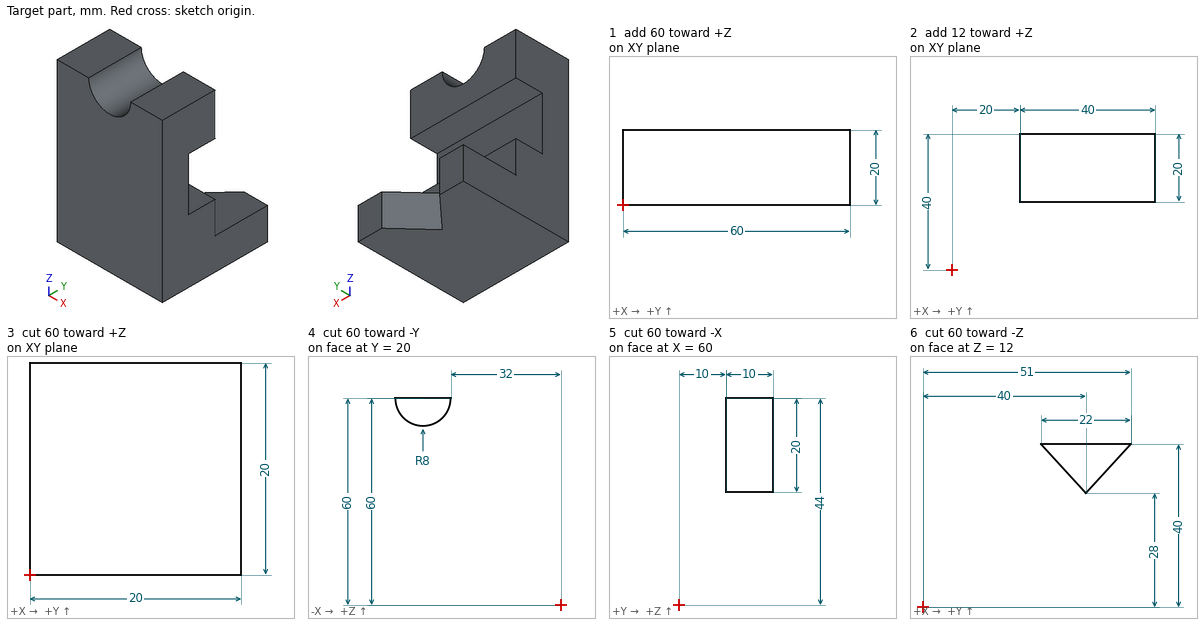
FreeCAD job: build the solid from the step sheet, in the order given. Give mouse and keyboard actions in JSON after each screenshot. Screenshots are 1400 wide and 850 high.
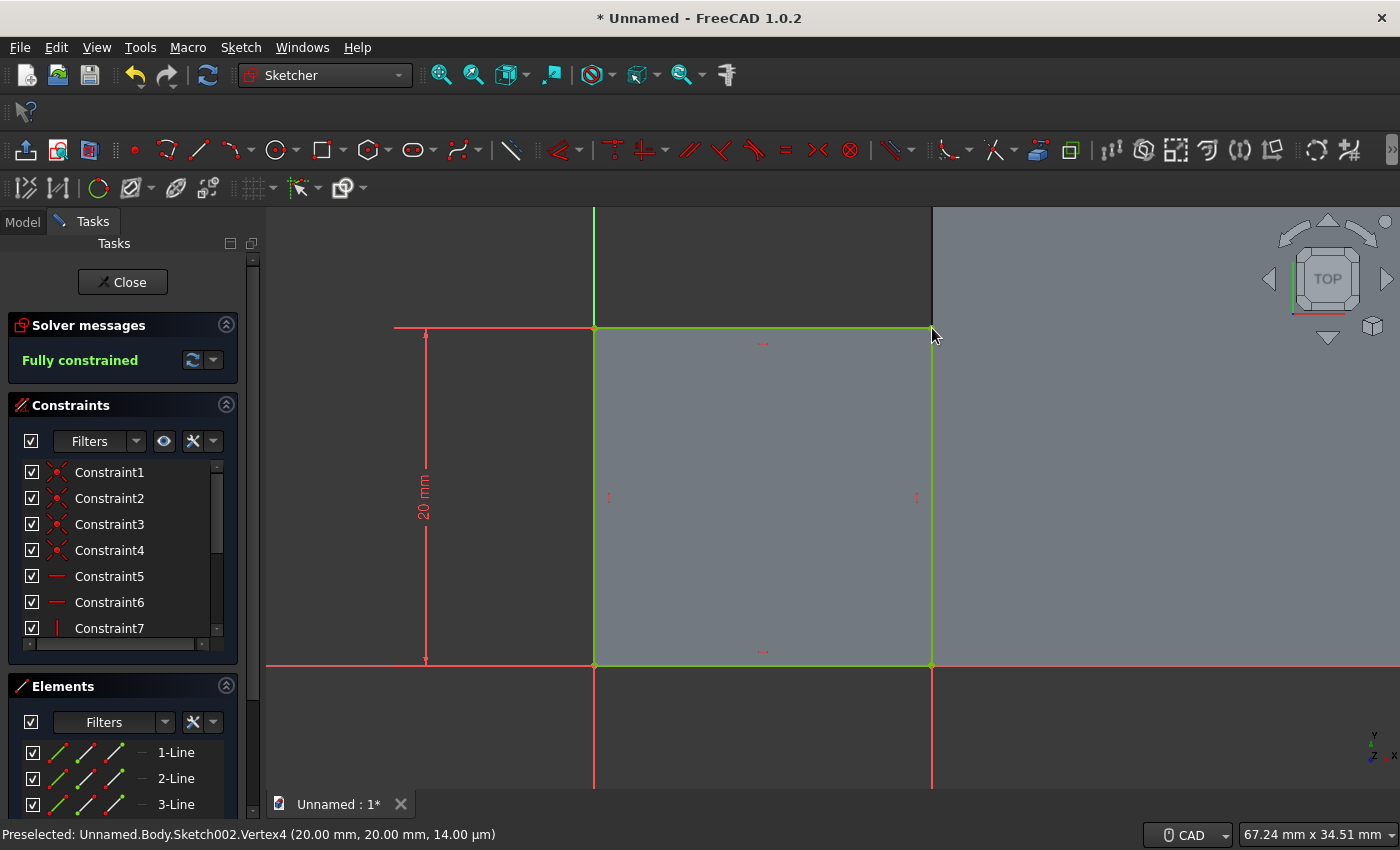
{"action": "left_click", "coordinate": [123, 282]}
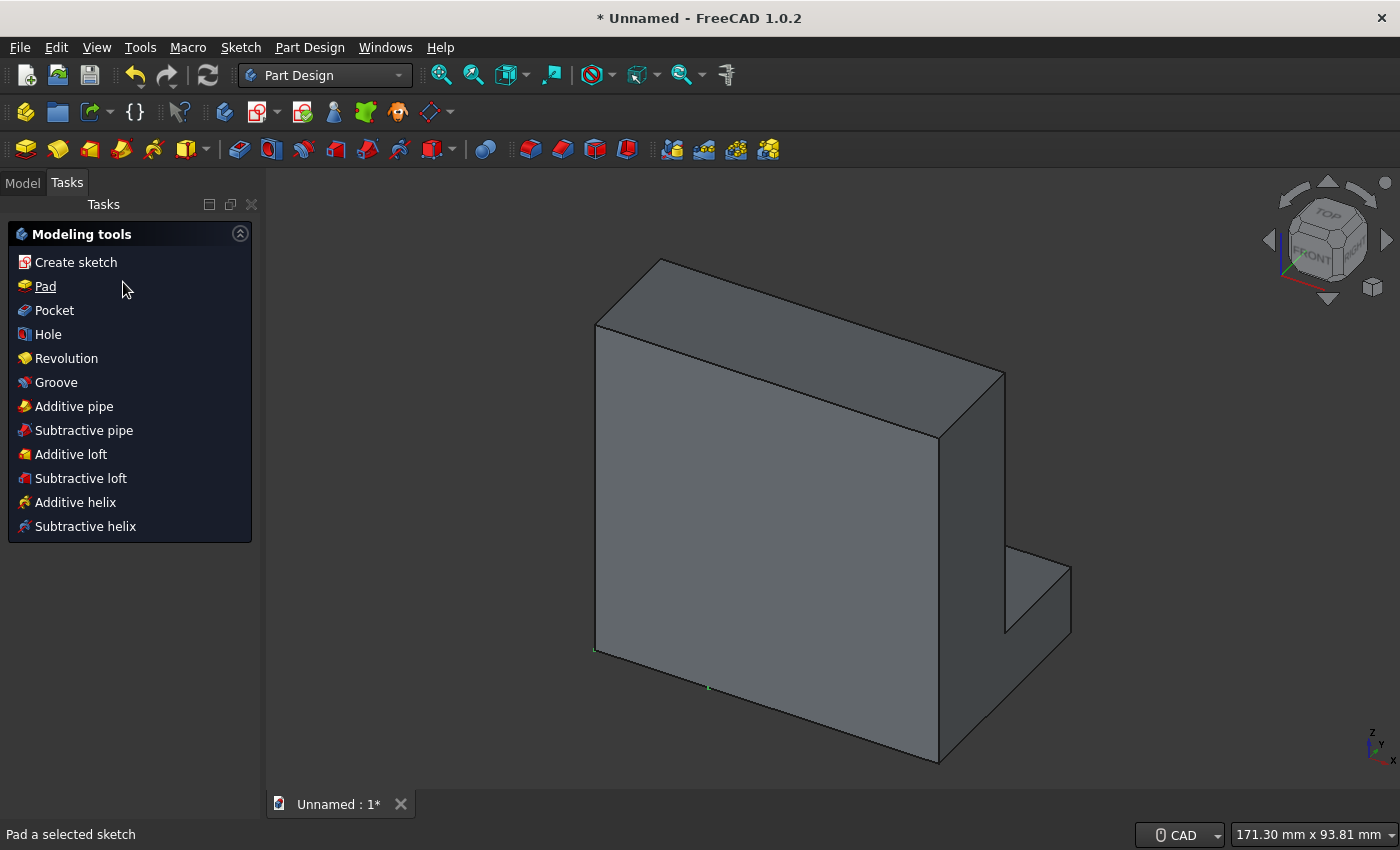
{"action": "left_click", "coordinate": [240, 150]}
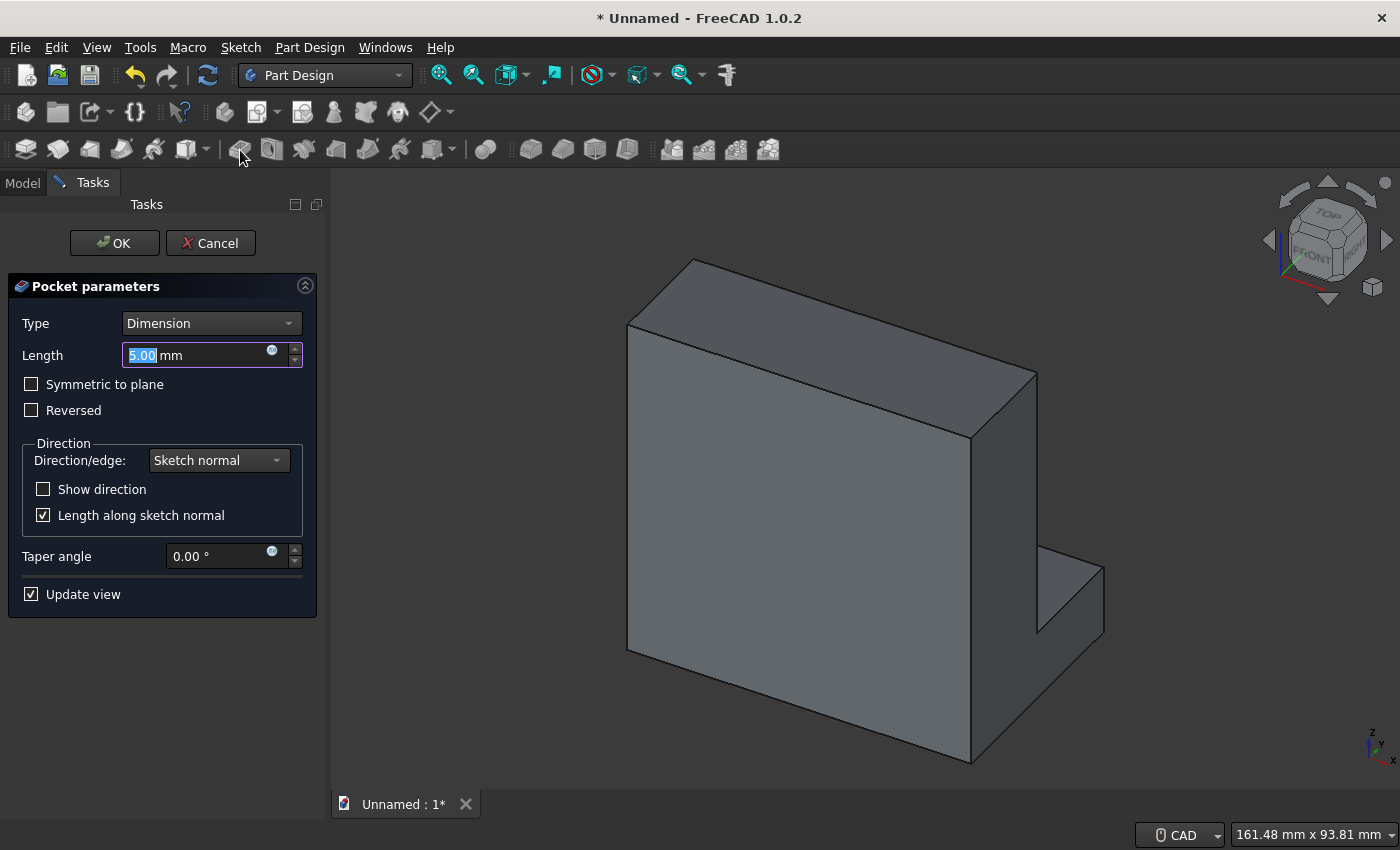
{"action": "type", "text": "60"}
{"action": "key", "text": "Tab"}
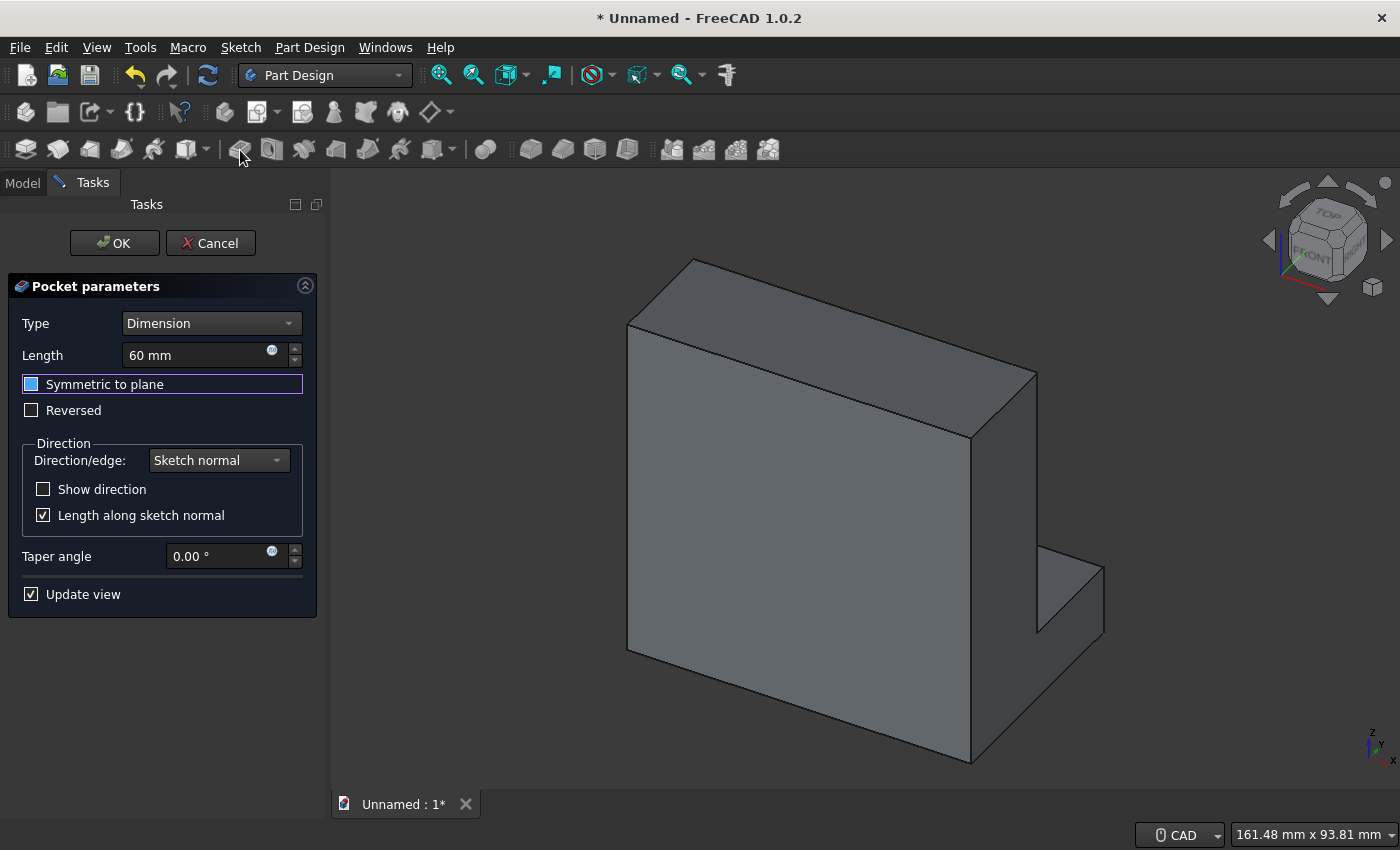
{"action": "left_click", "coordinate": [30, 410]}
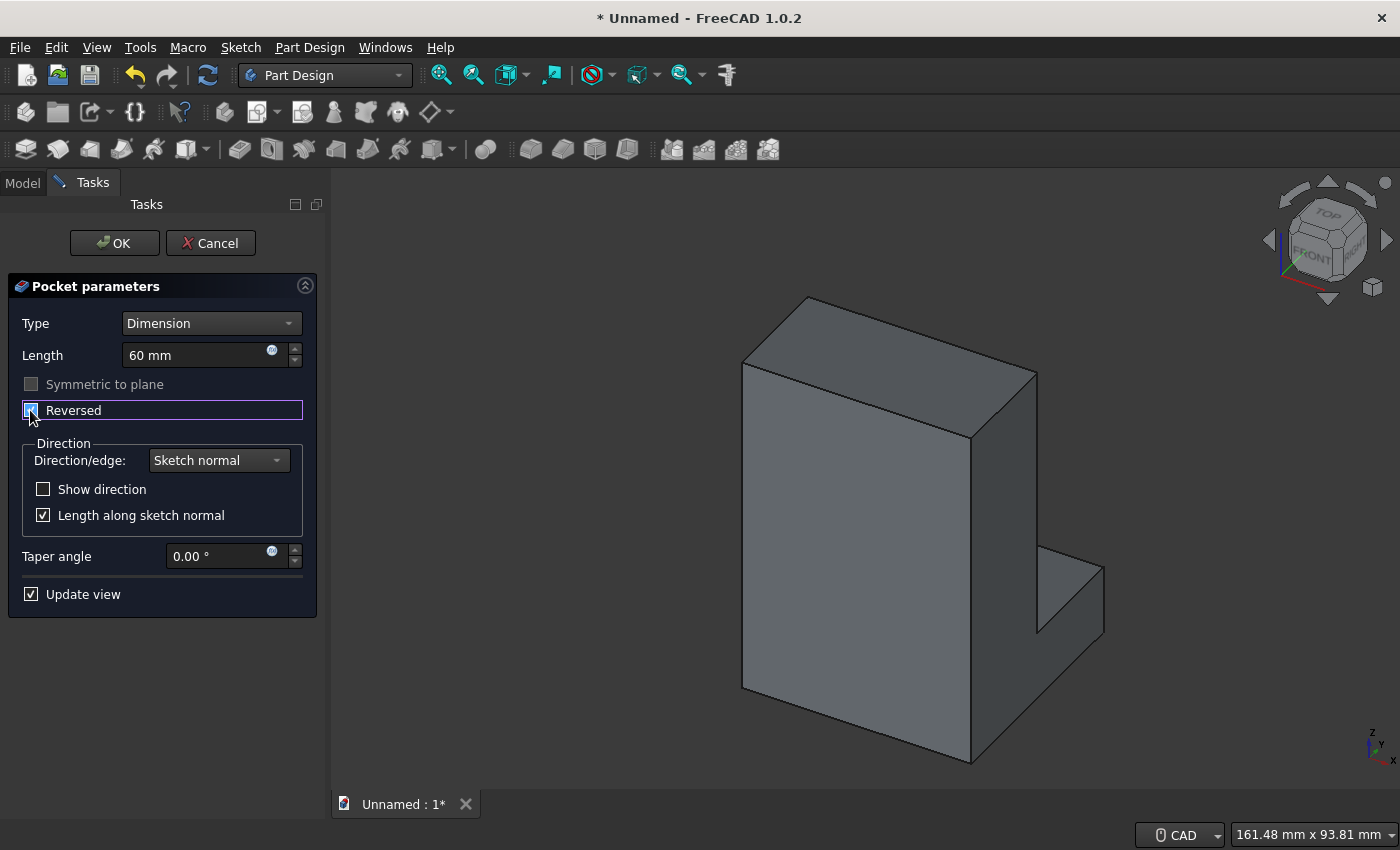
{"action": "left_click", "coordinate": [115, 243]}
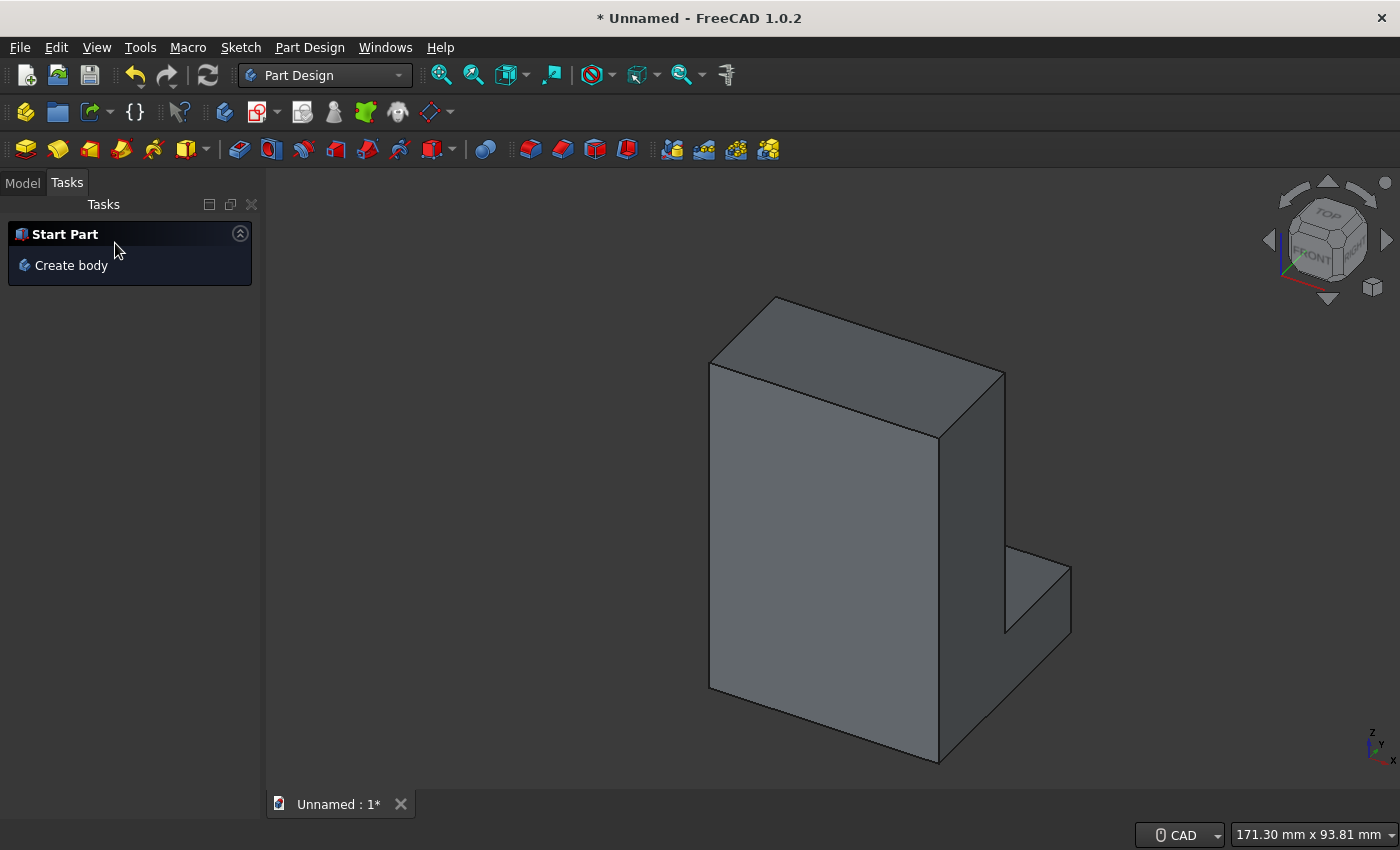
{"action": "key", "text": "4"}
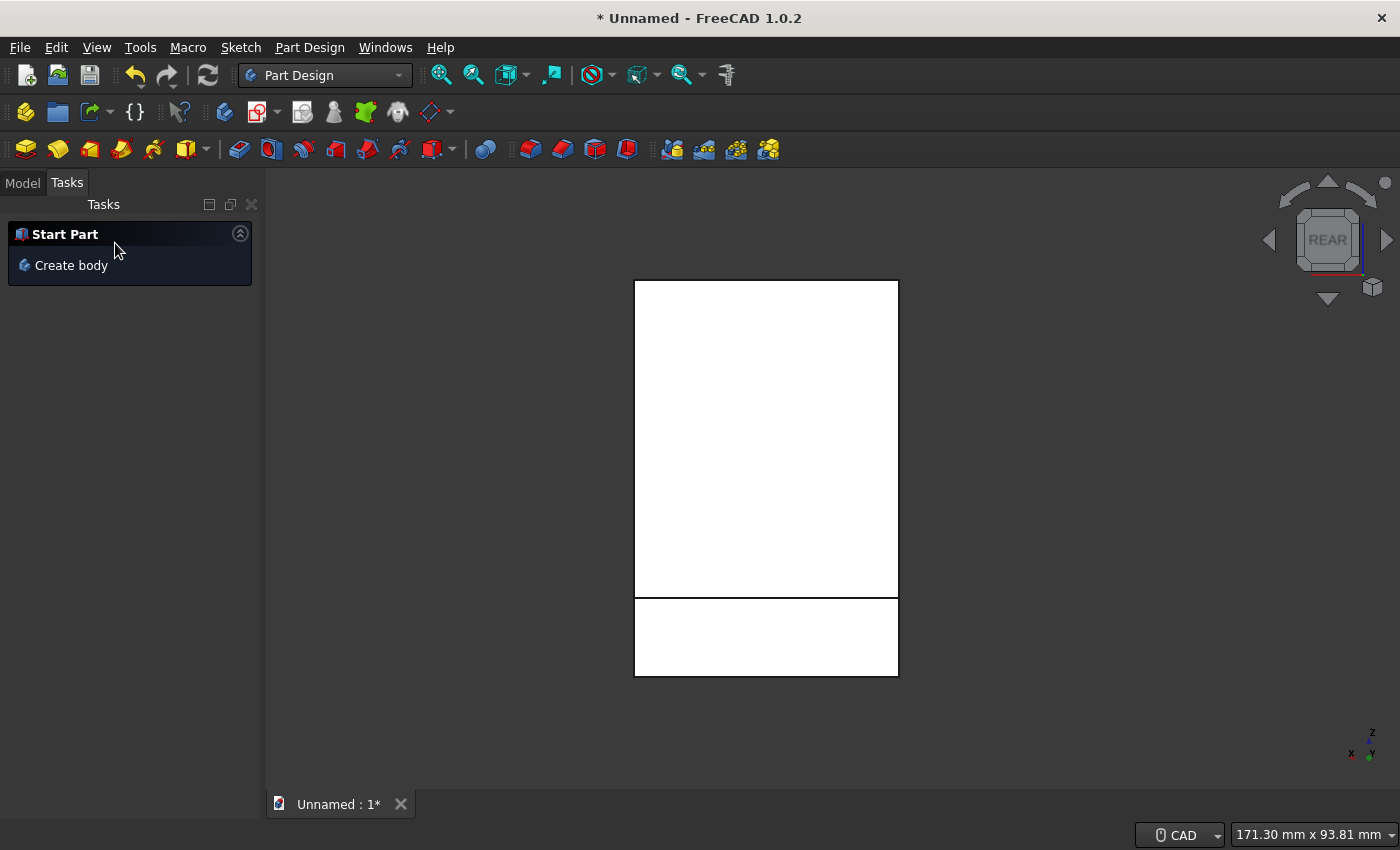
{"action": "left_click", "coordinate": [767, 438]}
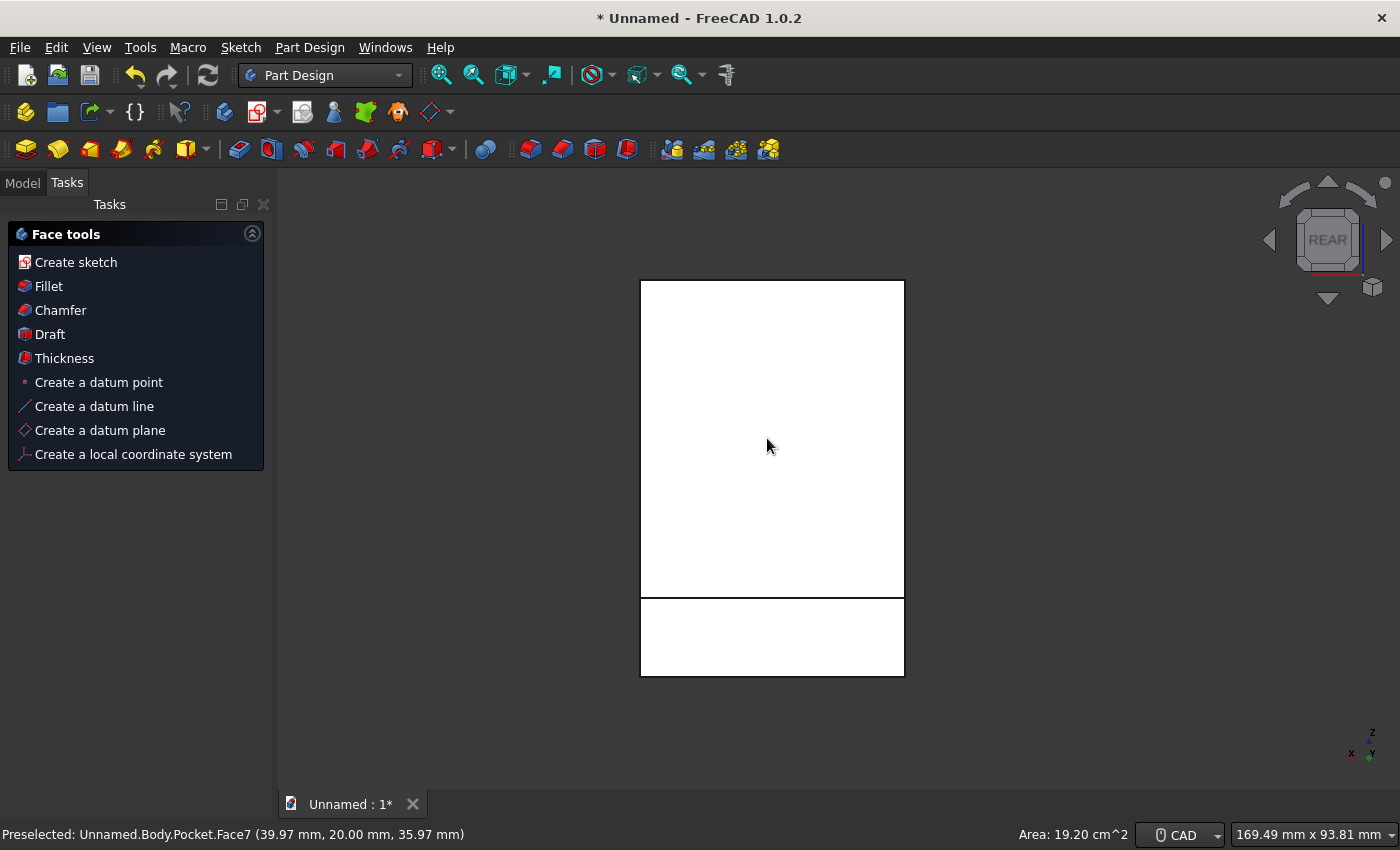
{"action": "left_click", "coordinate": [258, 112]}